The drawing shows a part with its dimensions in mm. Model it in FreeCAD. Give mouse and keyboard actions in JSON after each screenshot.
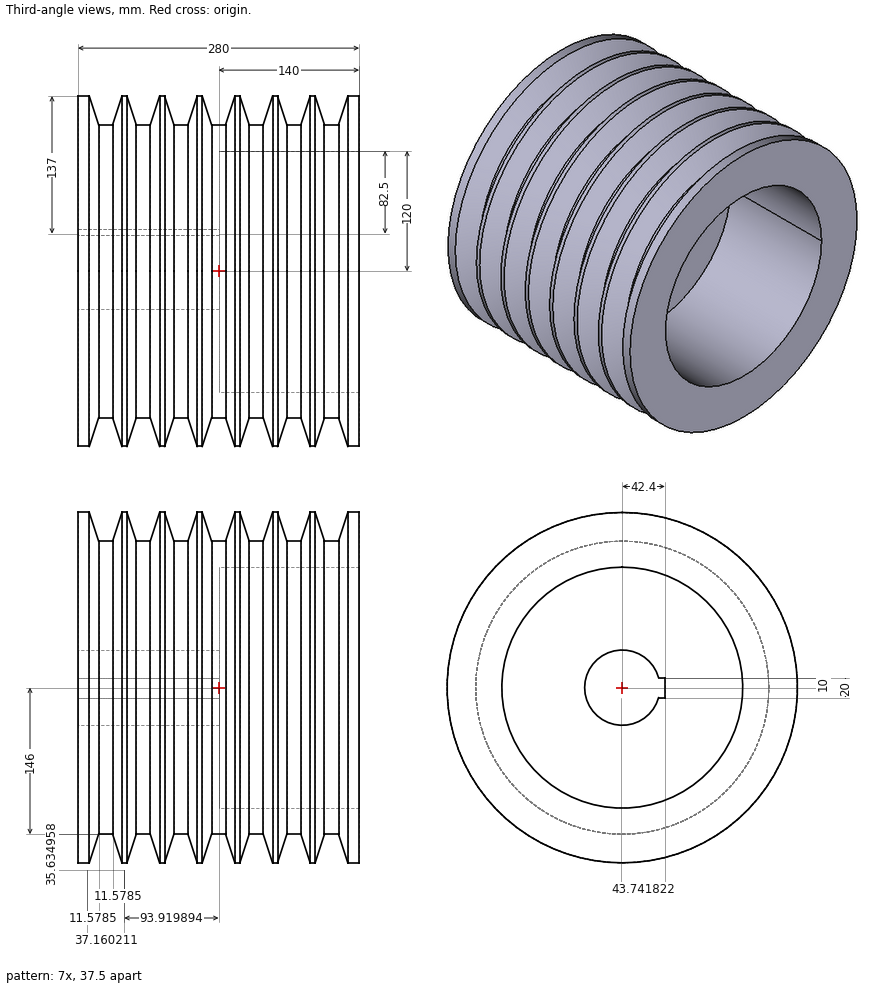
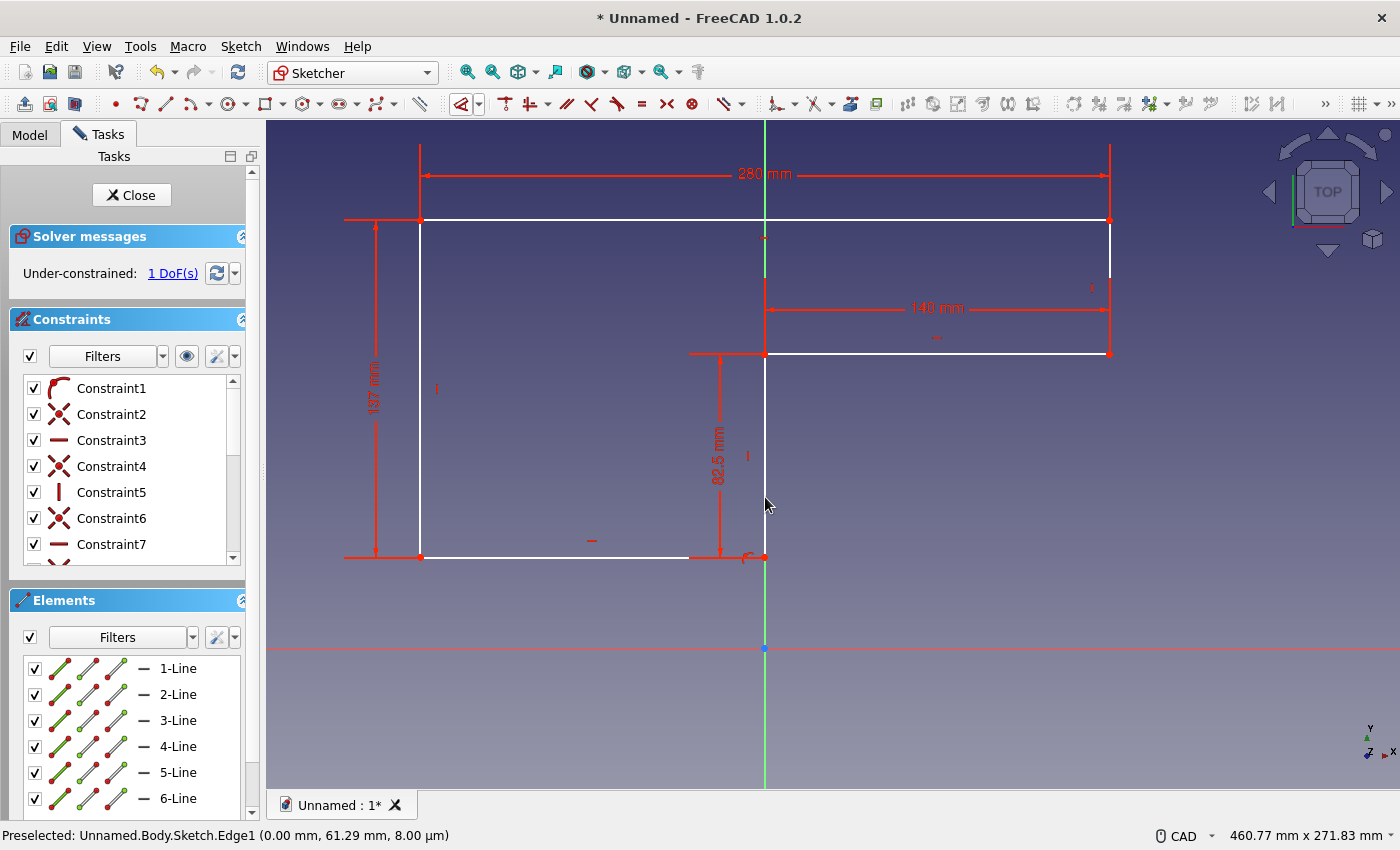
{"action": "left_click", "coordinate": [765, 354]}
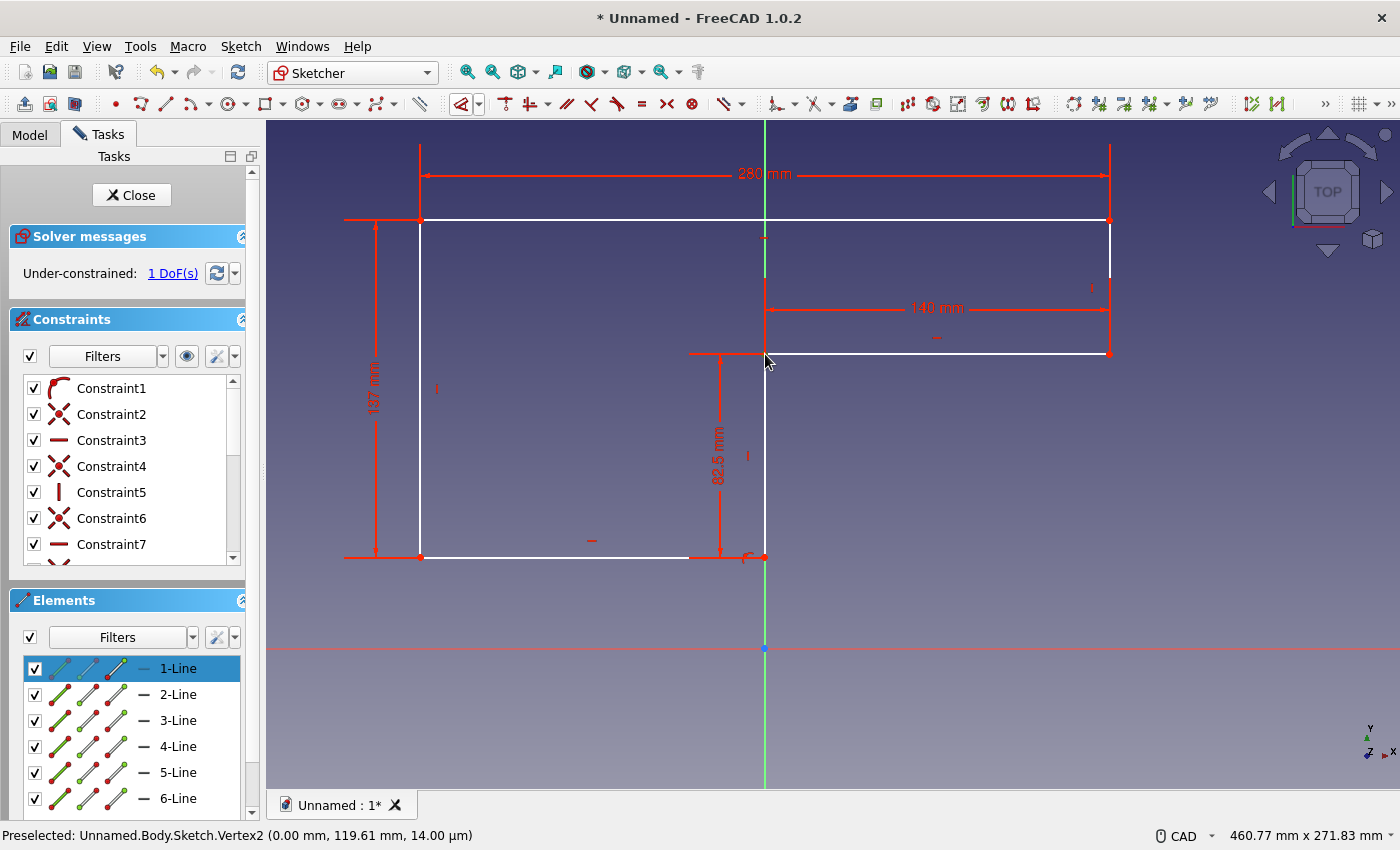
{"action": "key", "text": "i"}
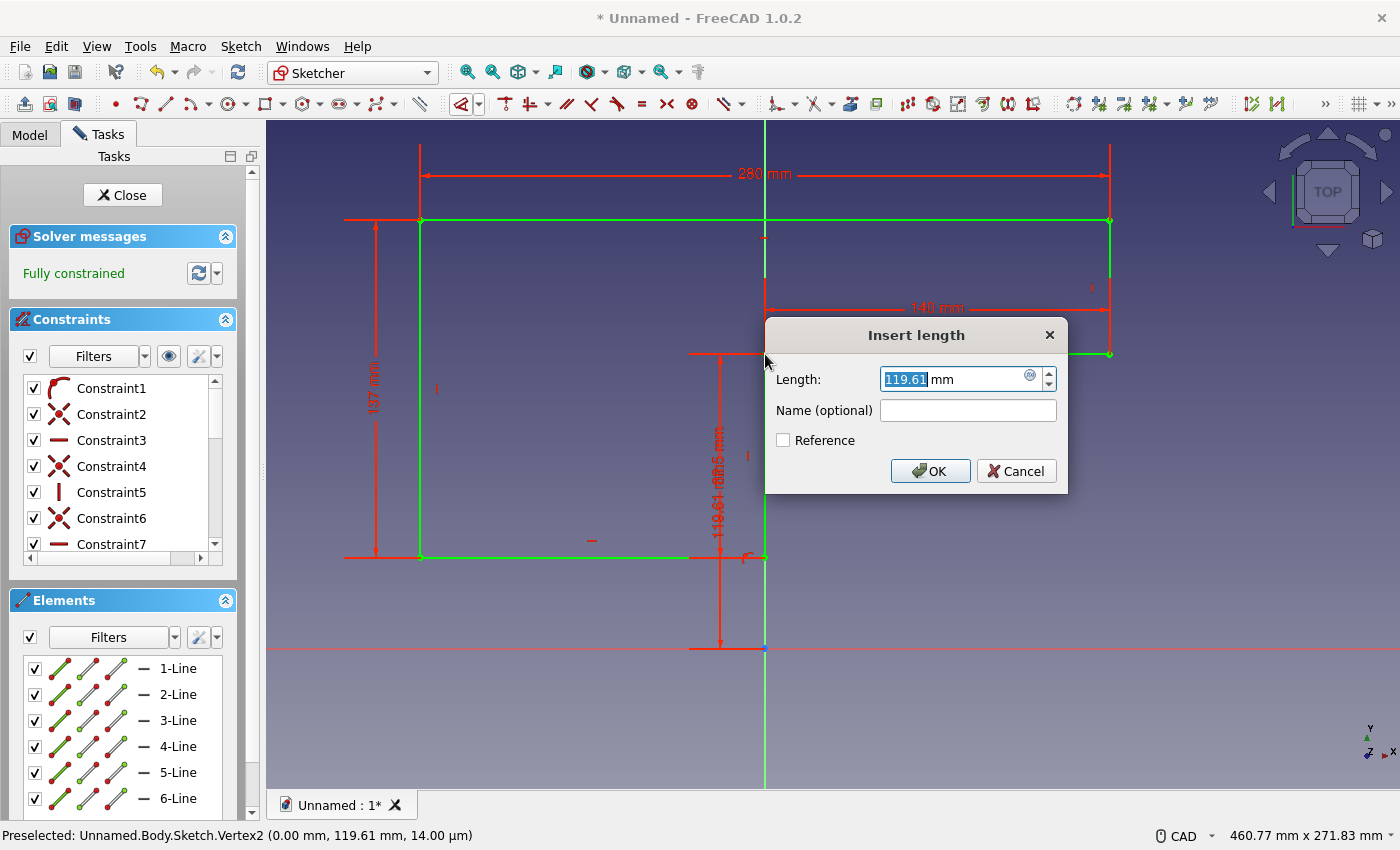
{"action": "type", "text": "120"}
{"action": "key", "text": "Return"}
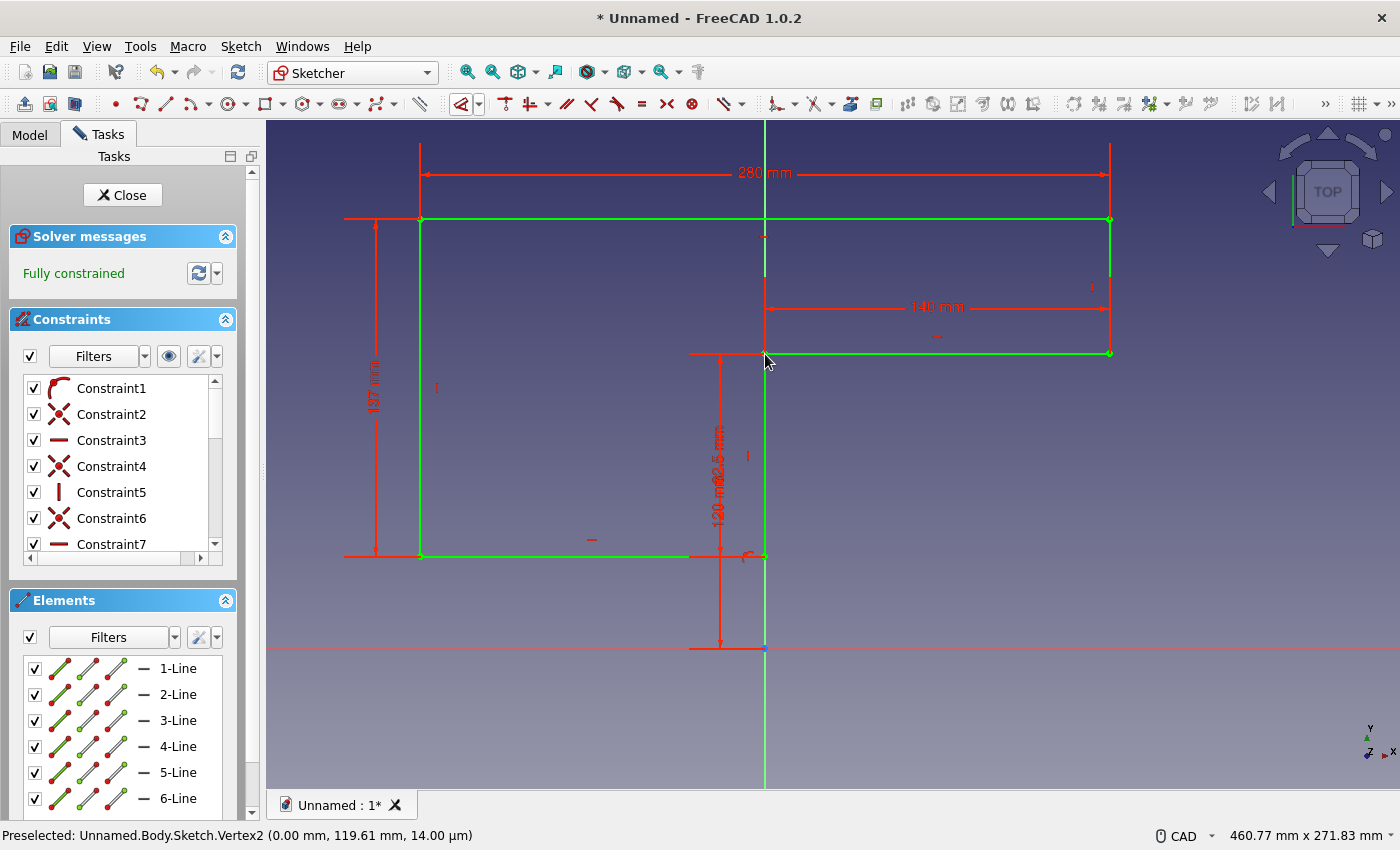
{"action": "left_click", "coordinate": [123, 195]}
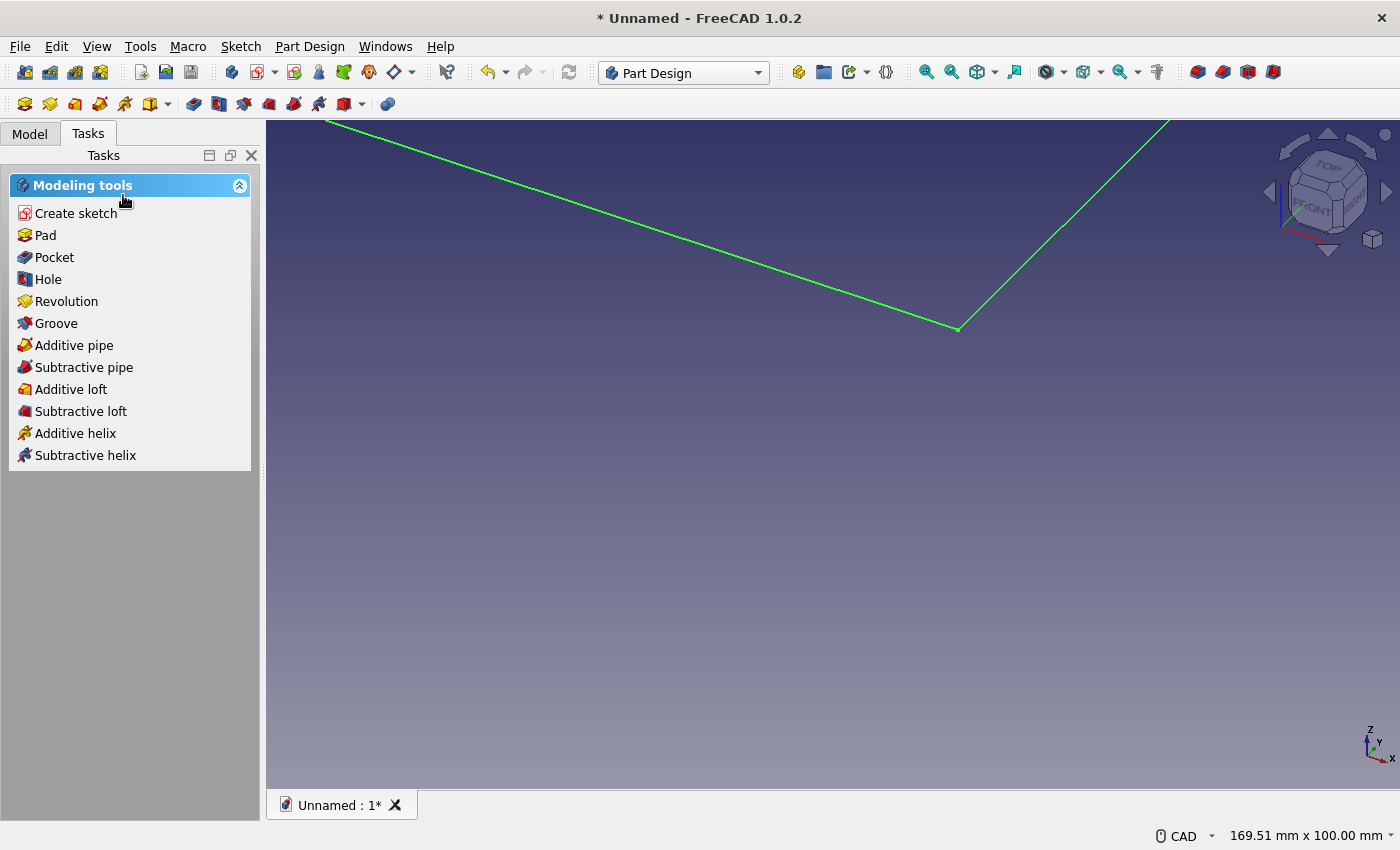
{"action": "left_click", "coordinate": [50, 104]}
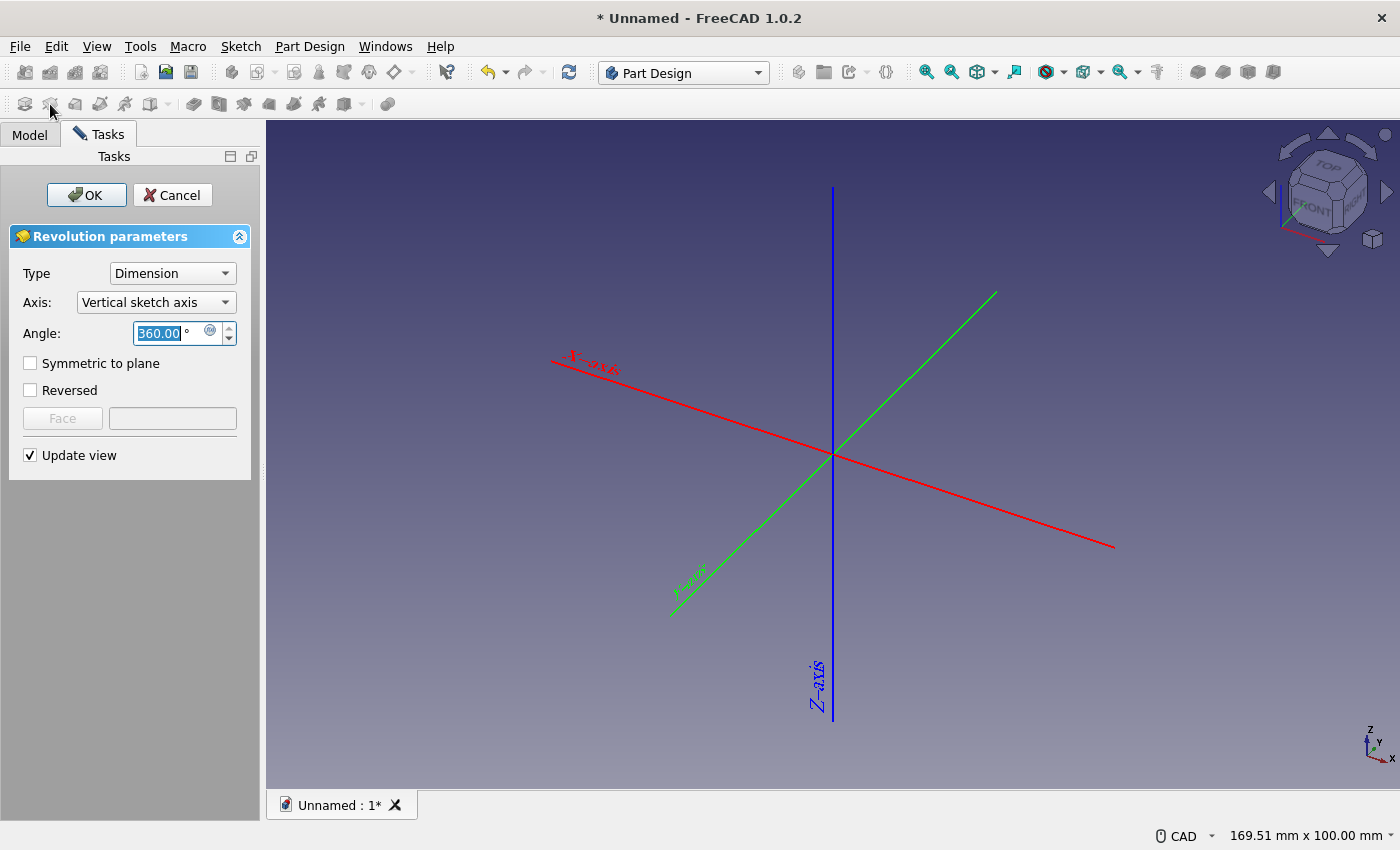
{"action": "left_click", "coordinate": [157, 302]}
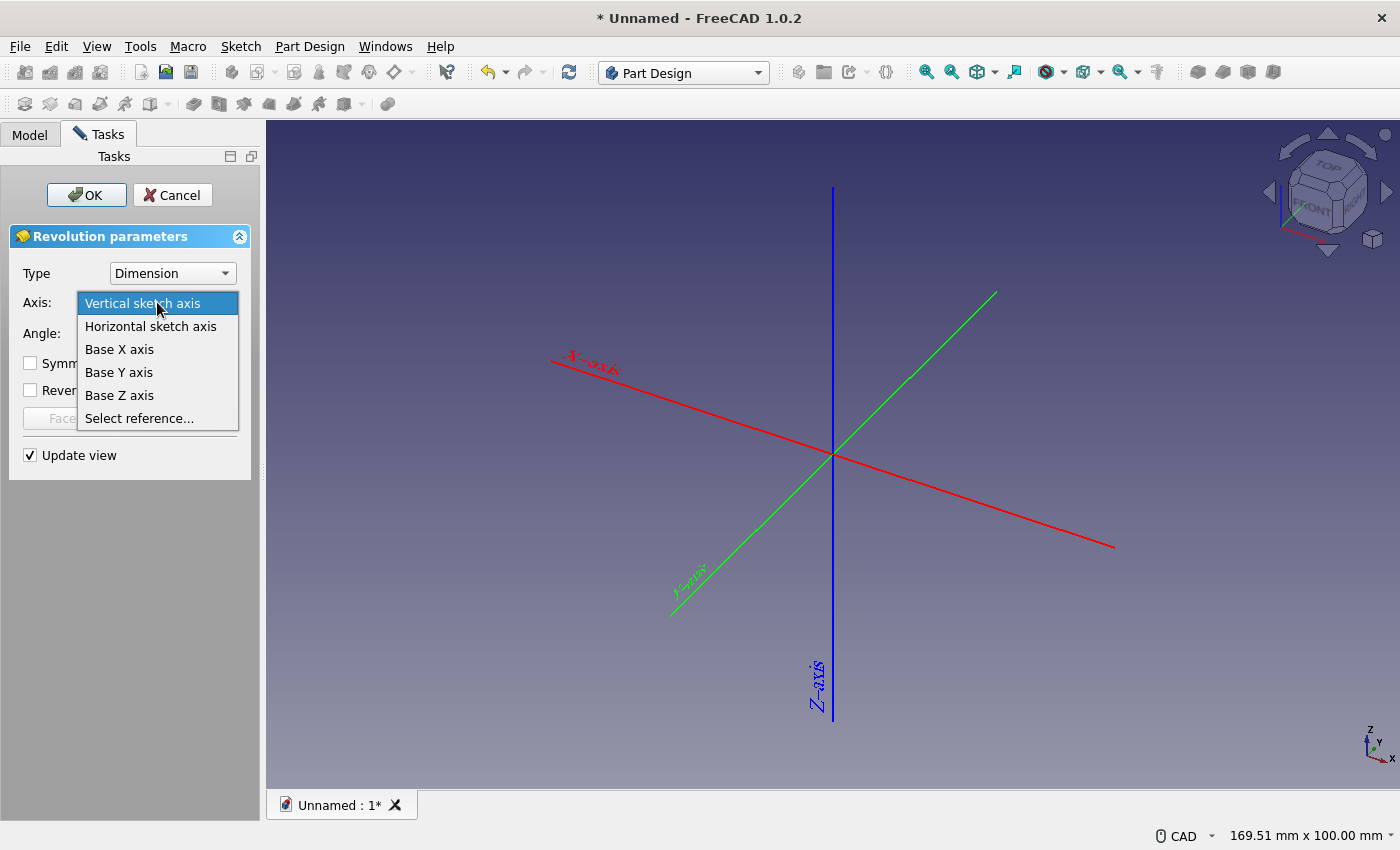
{"action": "left_click", "coordinate": [156, 326]}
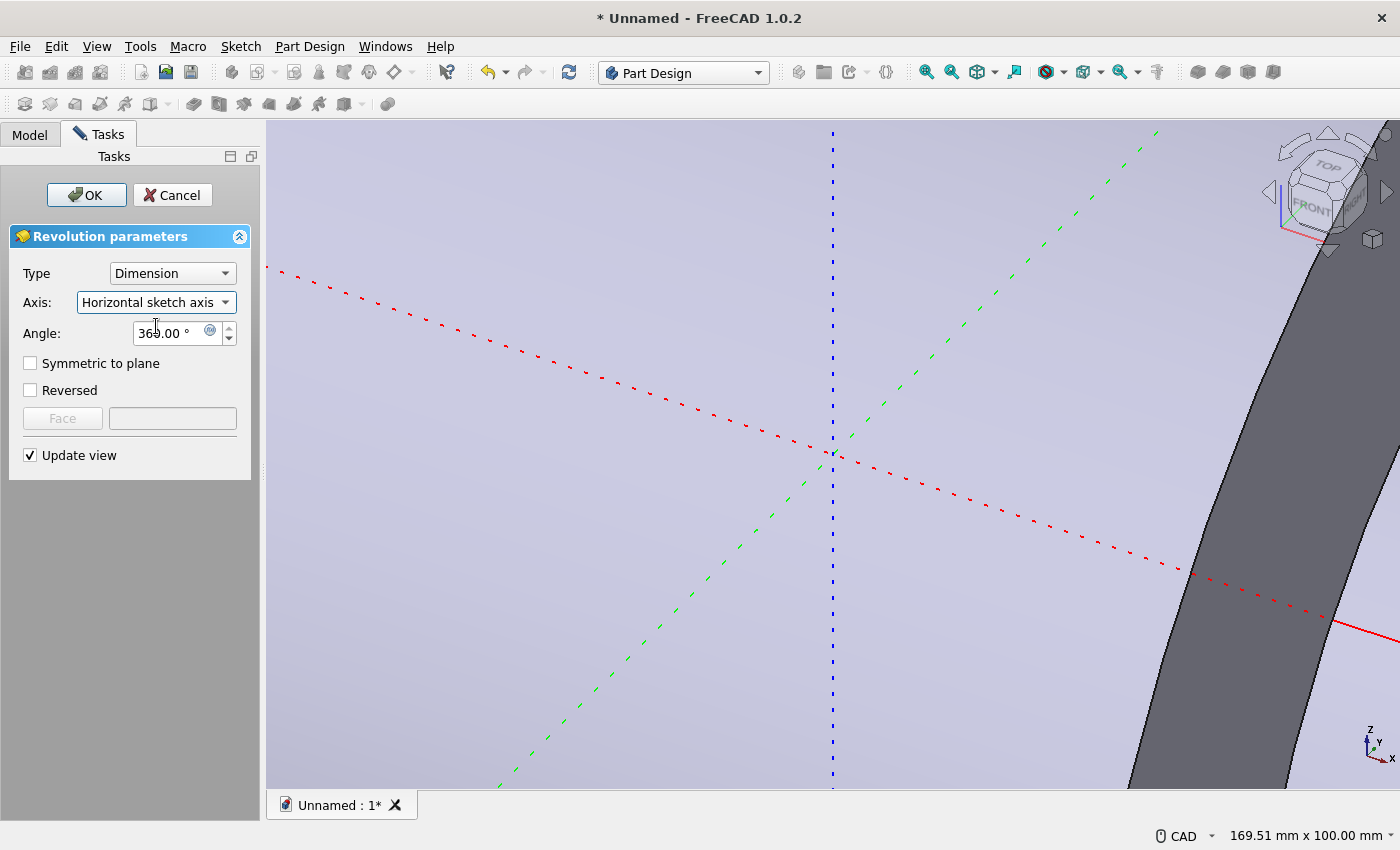
{"action": "left_click", "coordinate": [87, 195]}